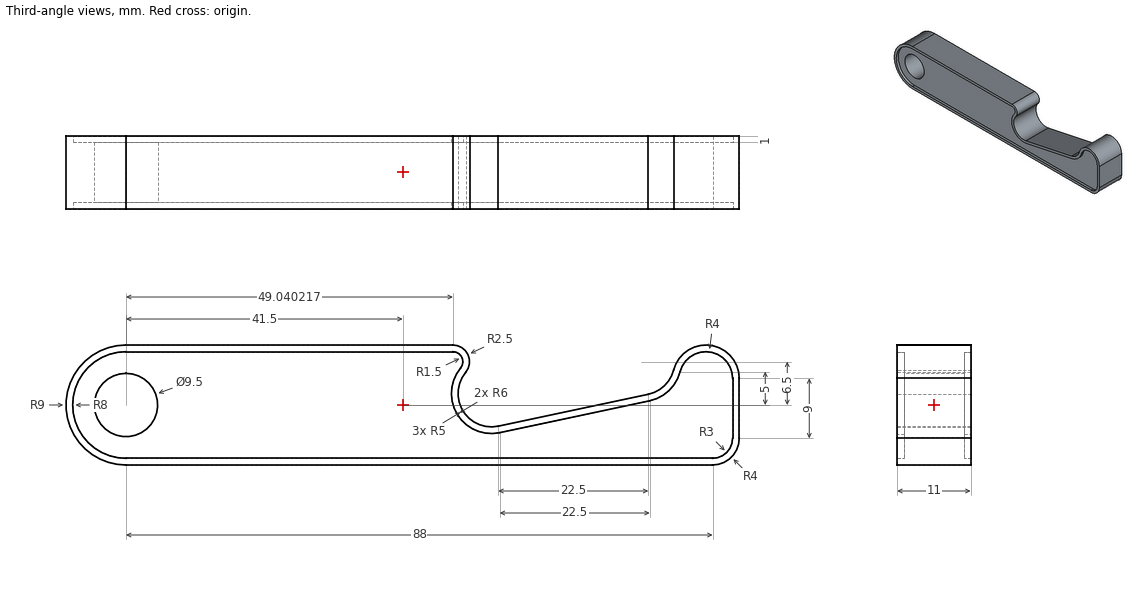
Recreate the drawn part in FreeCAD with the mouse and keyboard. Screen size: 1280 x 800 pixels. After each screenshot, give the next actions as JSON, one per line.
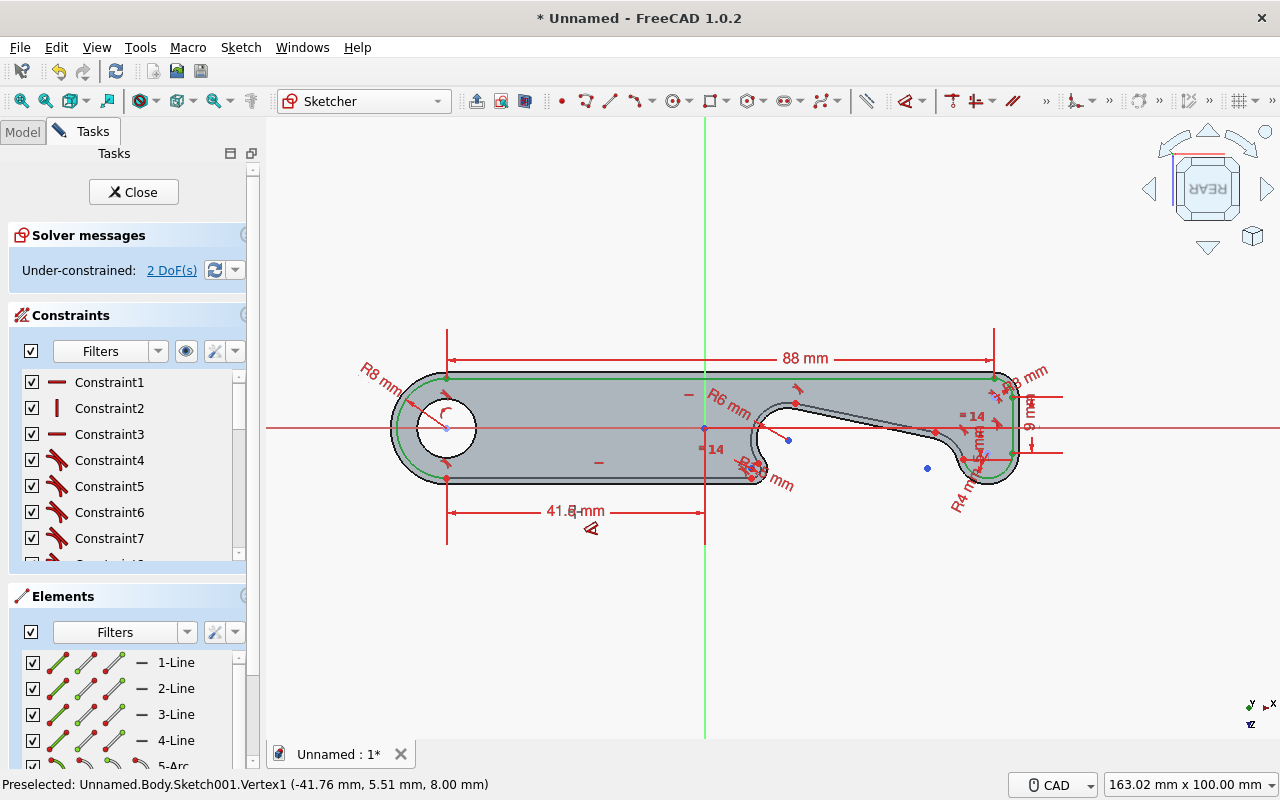
{"action": "left_click", "coordinate": [838, 412]}
{"action": "left_click", "coordinate": [865, 466]}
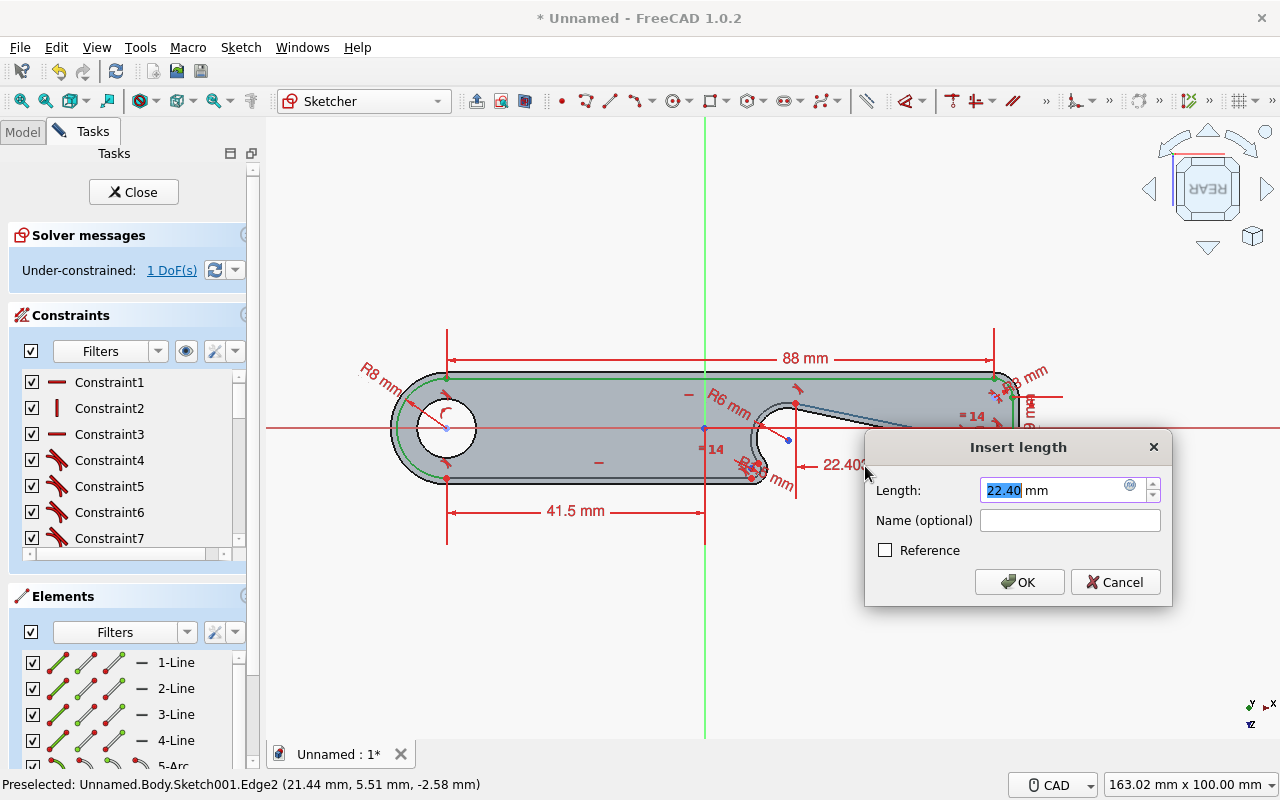
{"action": "type", "text": "22.5"}
{"action": "key", "text": "Return"}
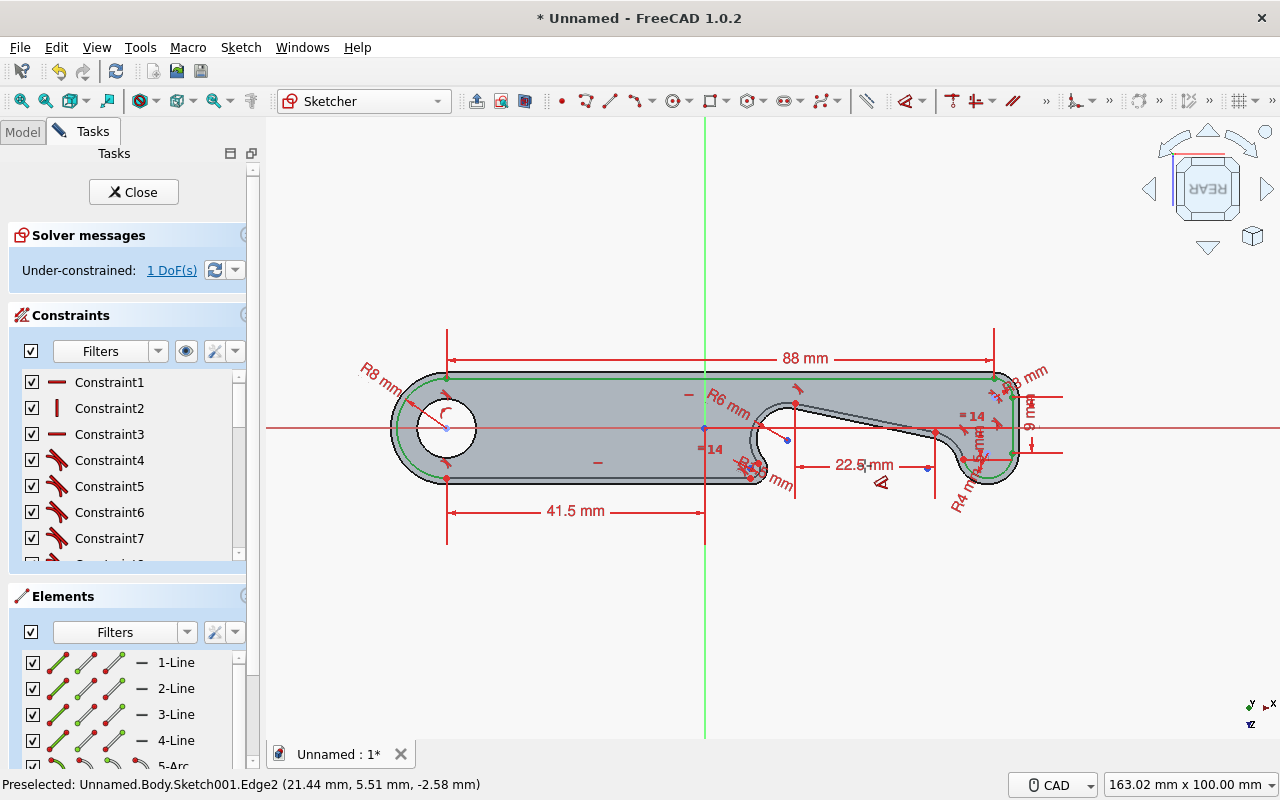
{"action": "left_click", "coordinate": [538, 478]}
{"action": "left_click", "coordinate": [669, 512]}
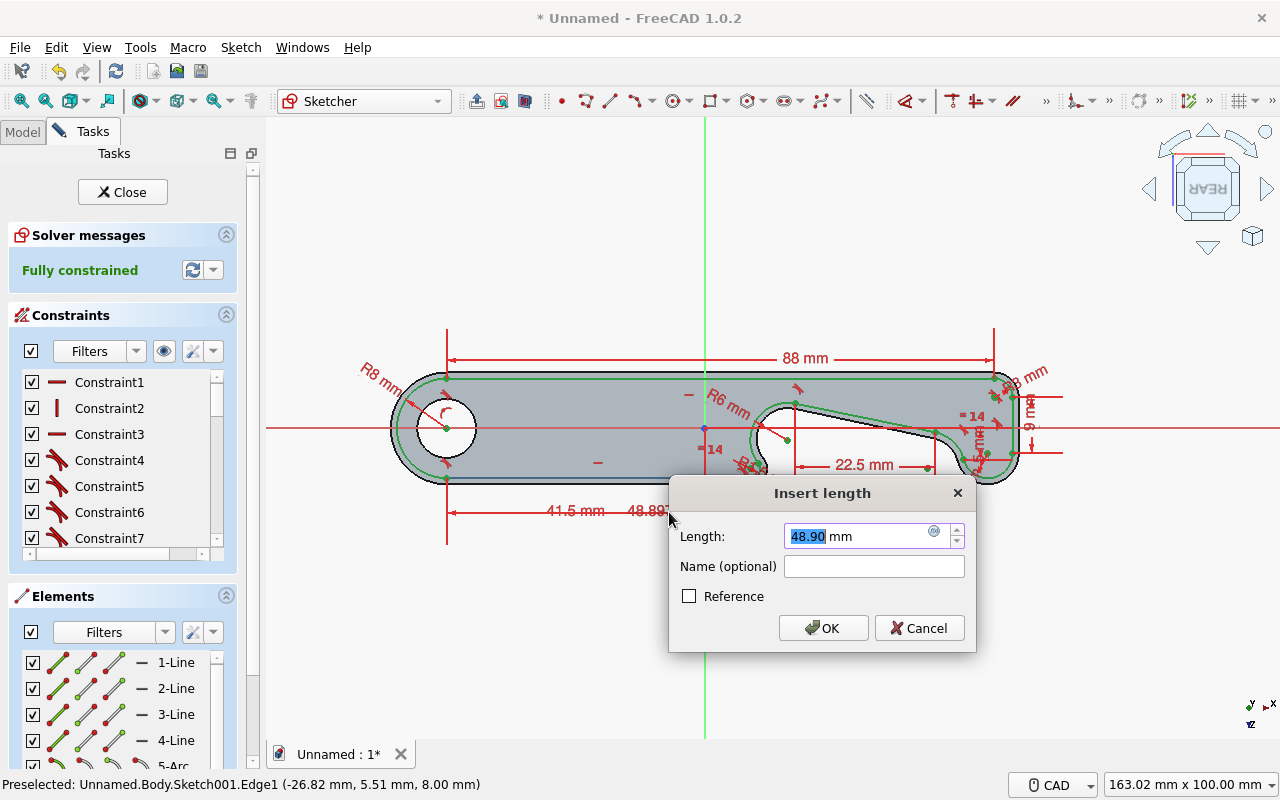
{"action": "type", "text": "49.040217"}
{"action": "key", "text": "Return"}
{"action": "key", "text": "Escape"}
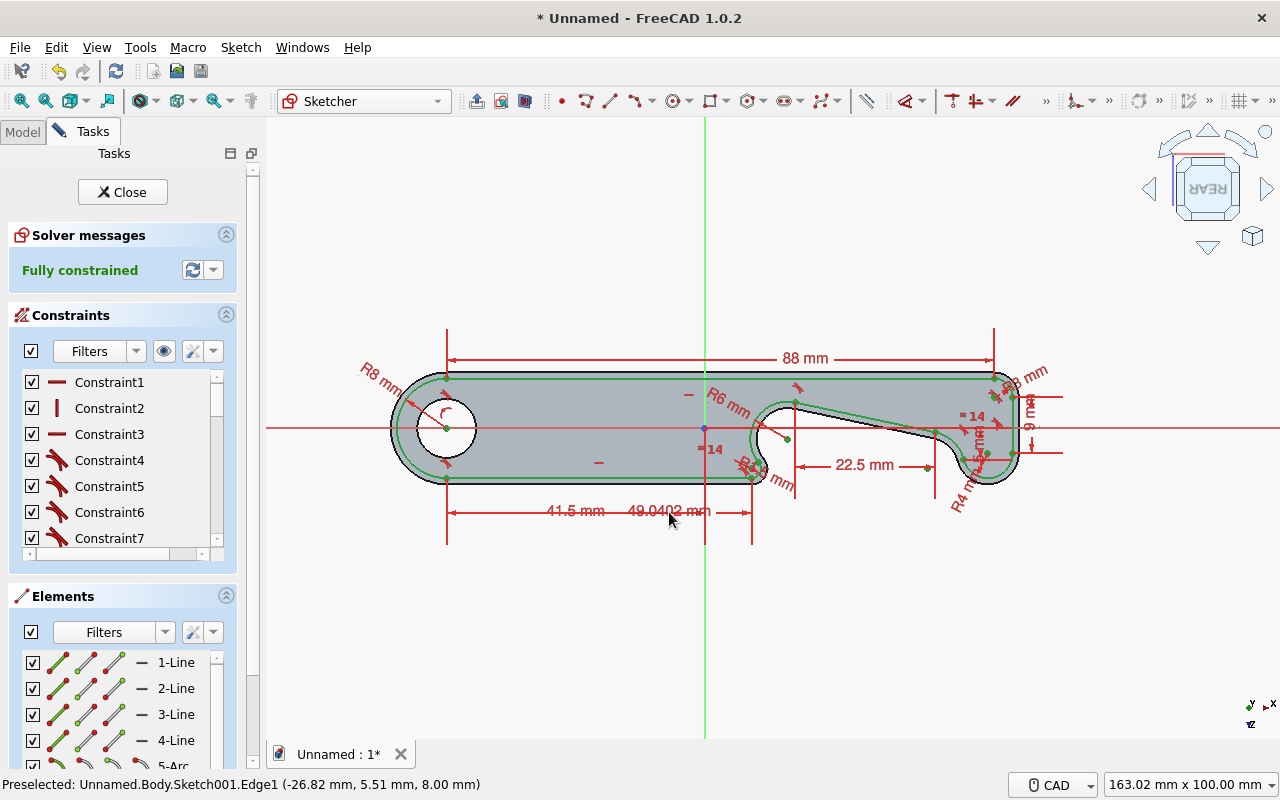
{"action": "left_click", "coordinate": [123, 192]}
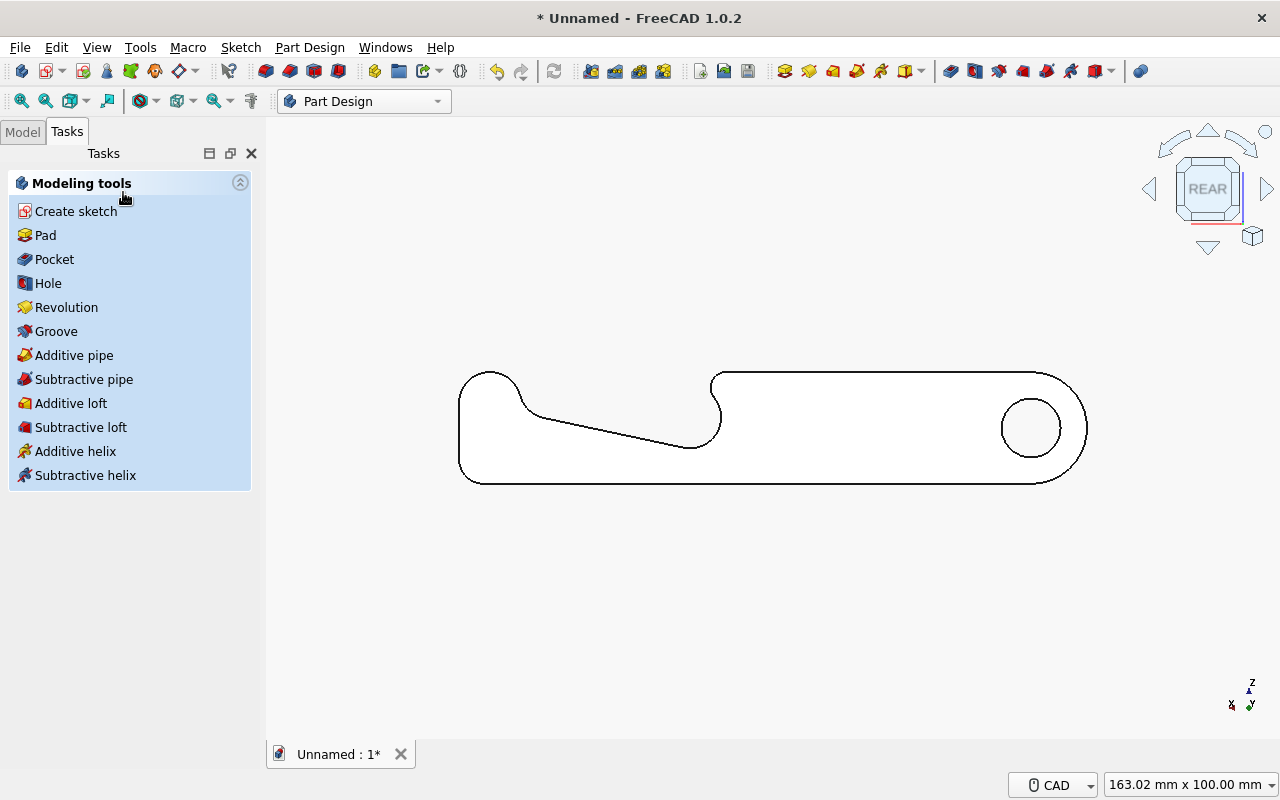
{"action": "left_click", "coordinate": [952, 72]}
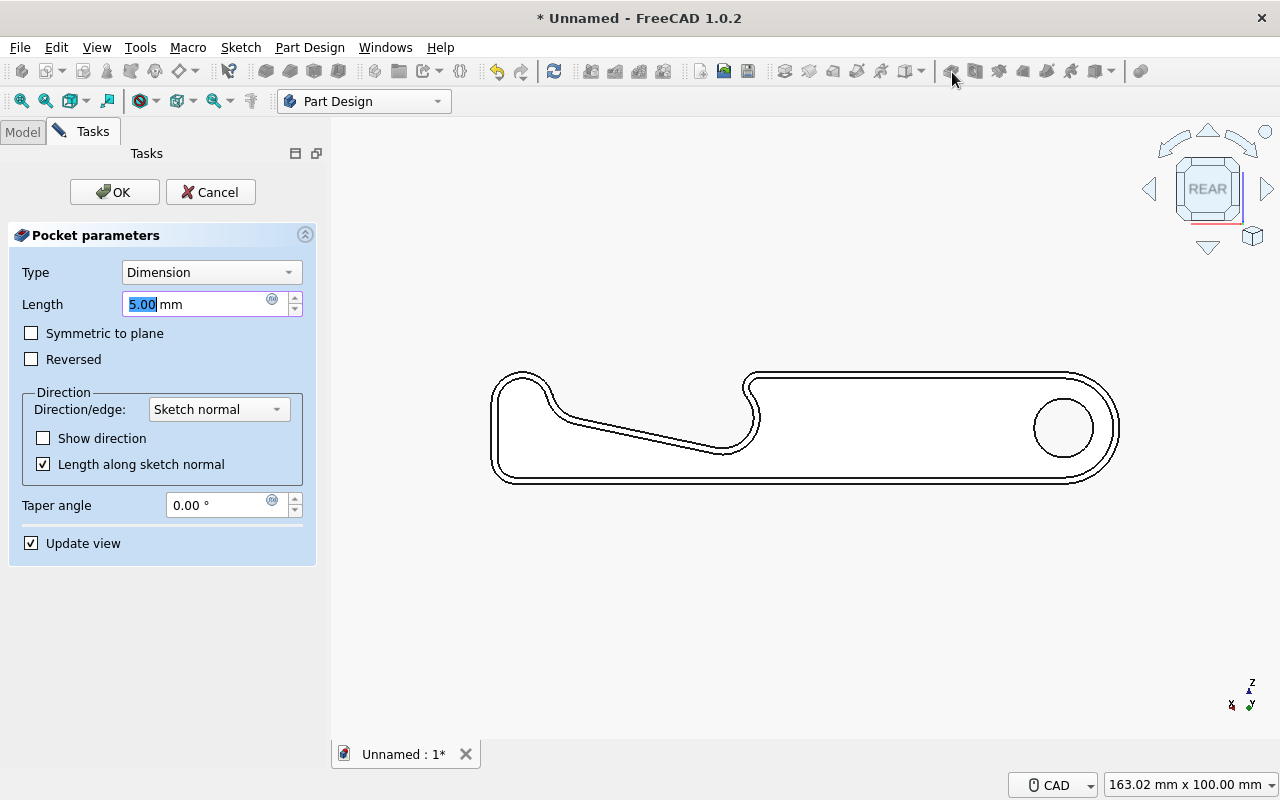
{"action": "type", "text": "1"}
{"action": "key", "text": "Tab"}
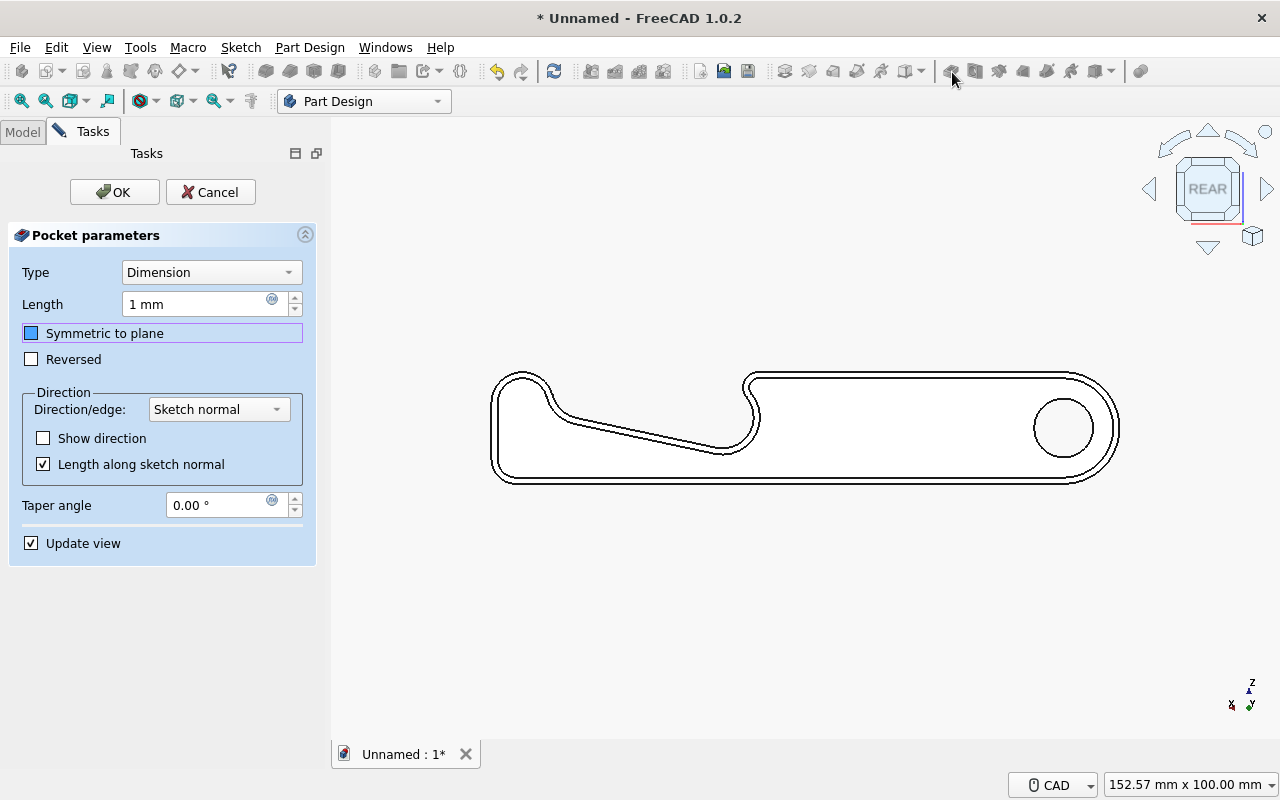
{"action": "left_click", "coordinate": [115, 192]}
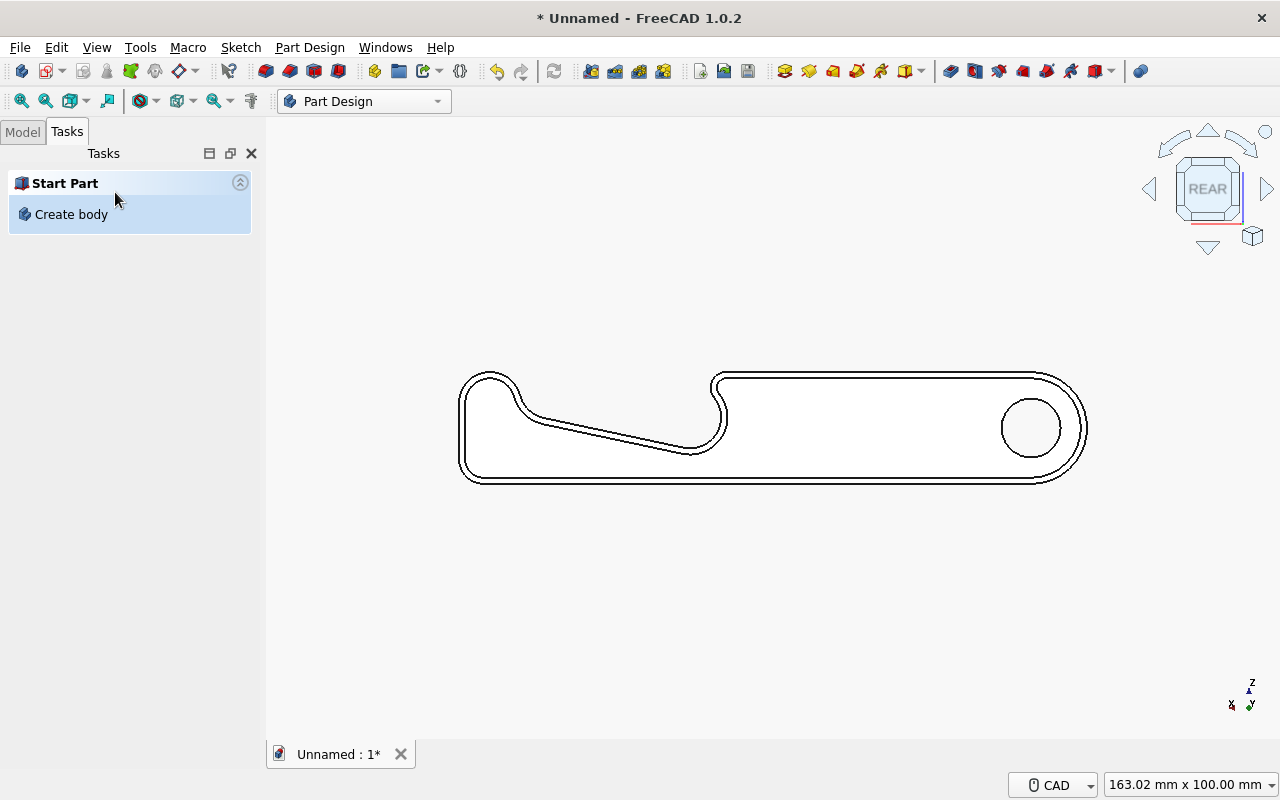
{"action": "left_click", "coordinate": [23, 131]}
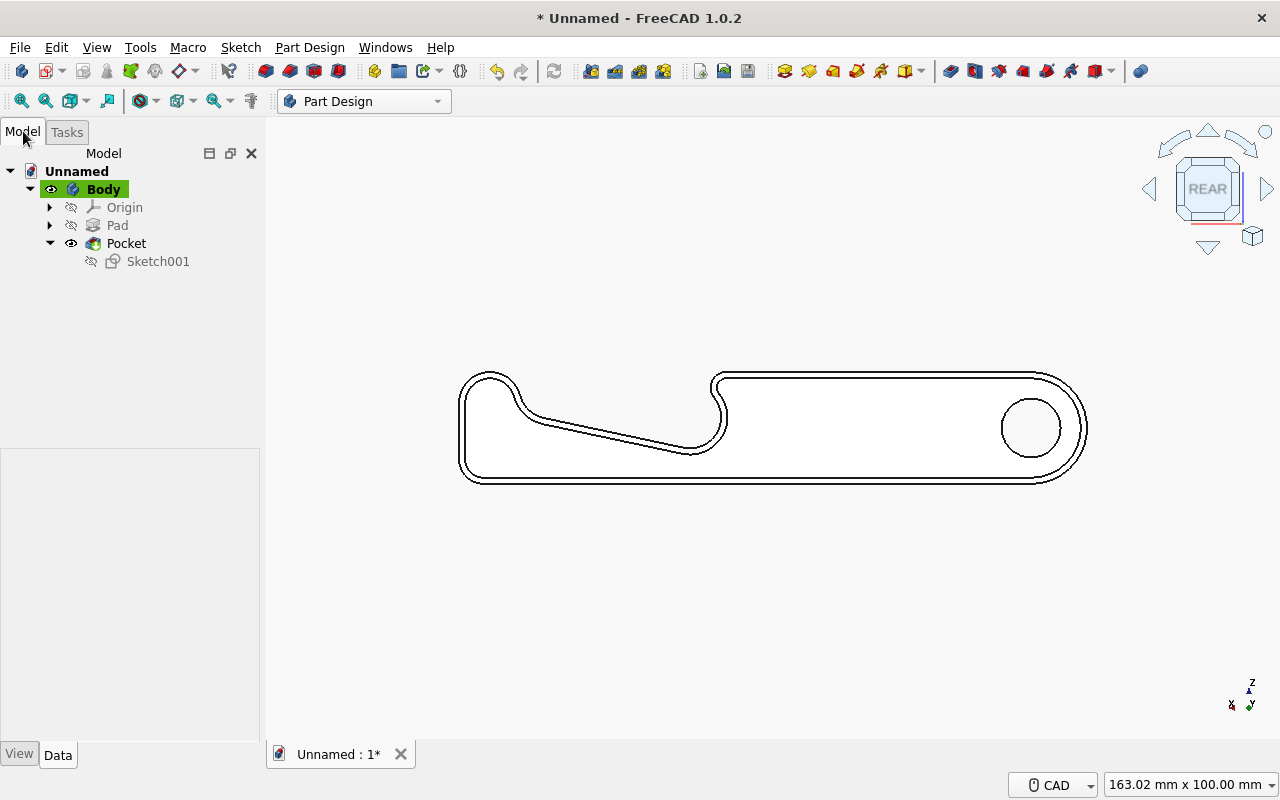
{"action": "left_click", "coordinate": [116, 243]}